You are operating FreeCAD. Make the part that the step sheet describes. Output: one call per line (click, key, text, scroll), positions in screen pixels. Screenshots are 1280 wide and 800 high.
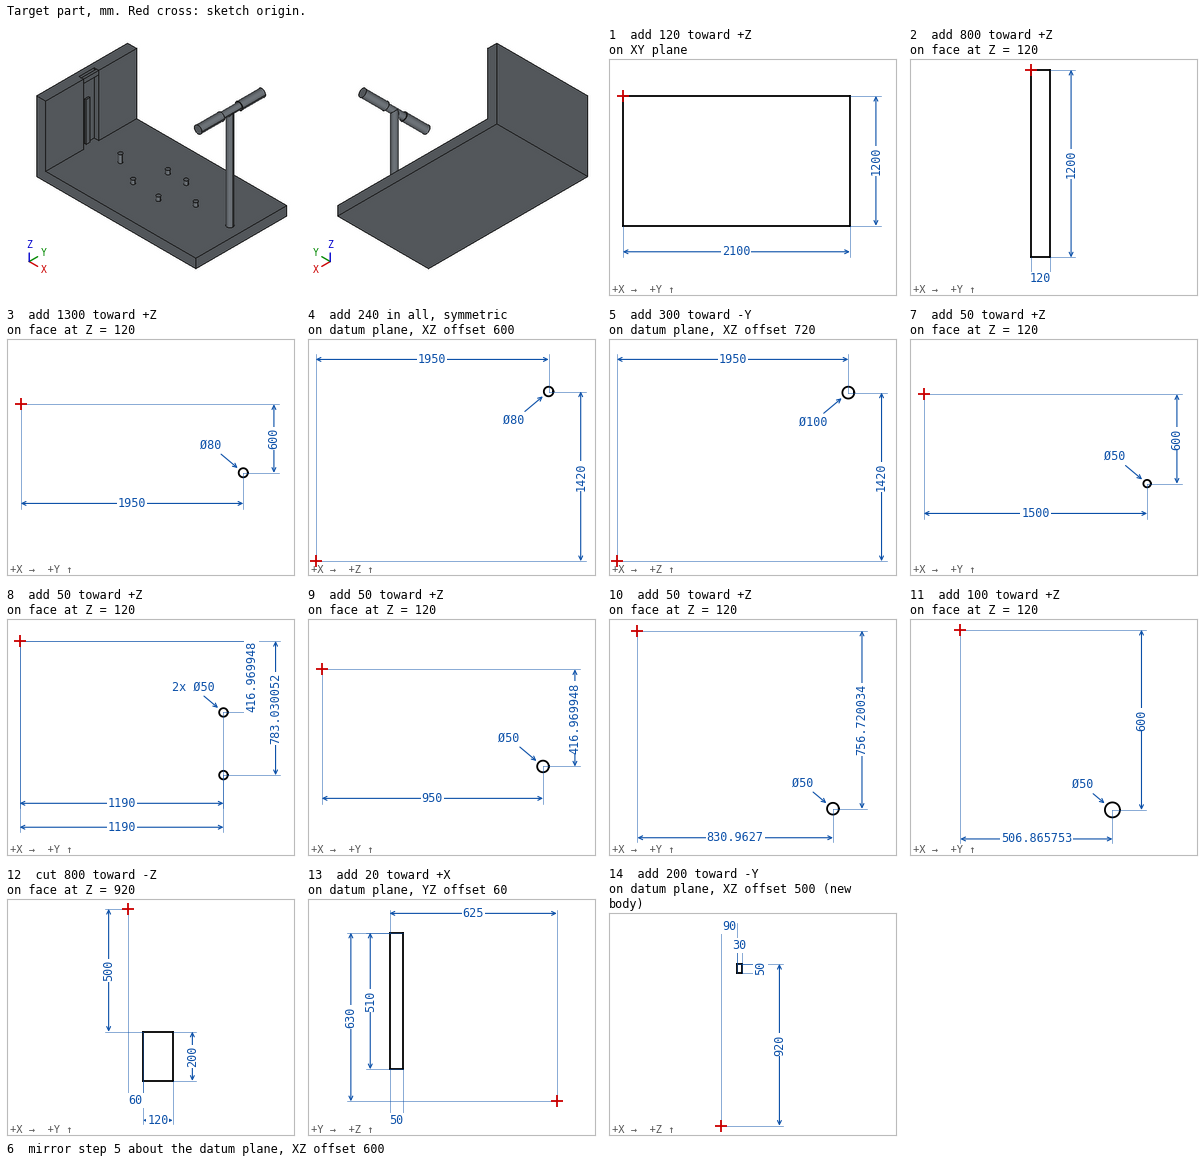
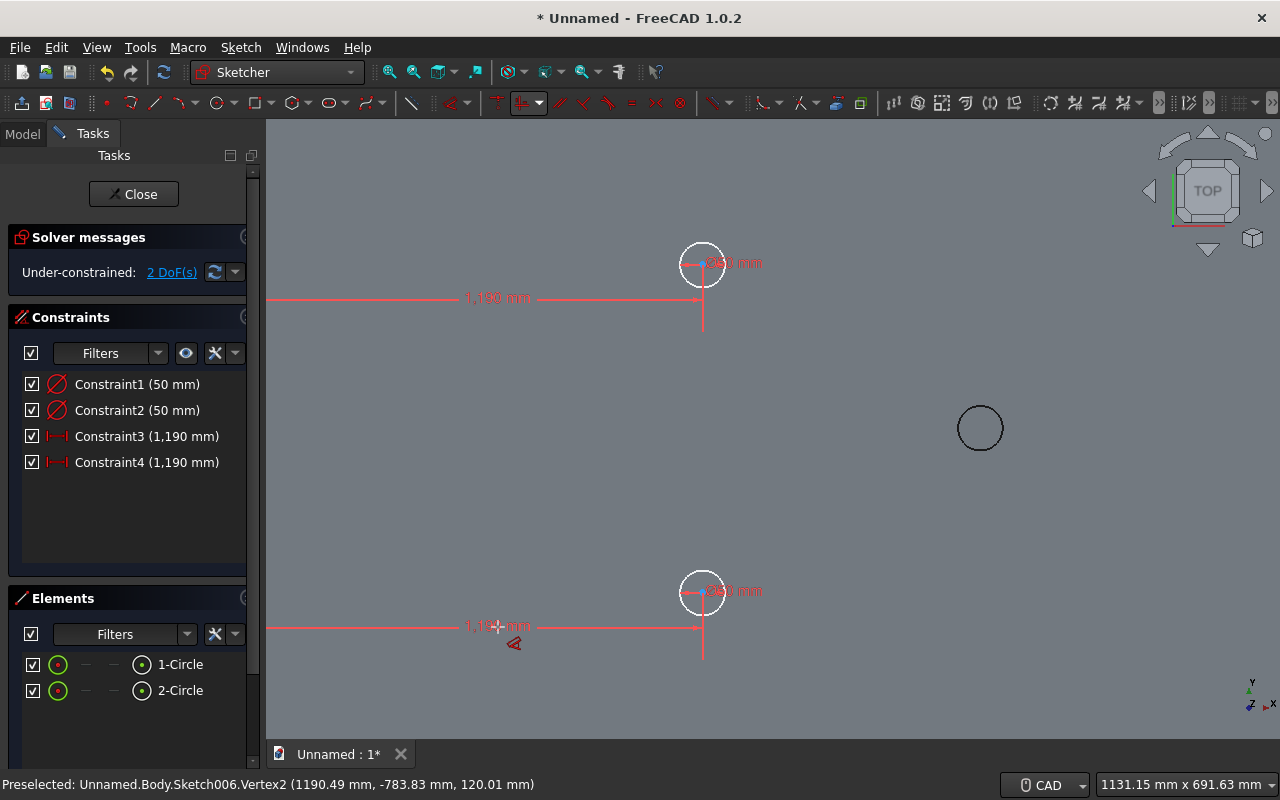
click(703, 265)
click(737, 206)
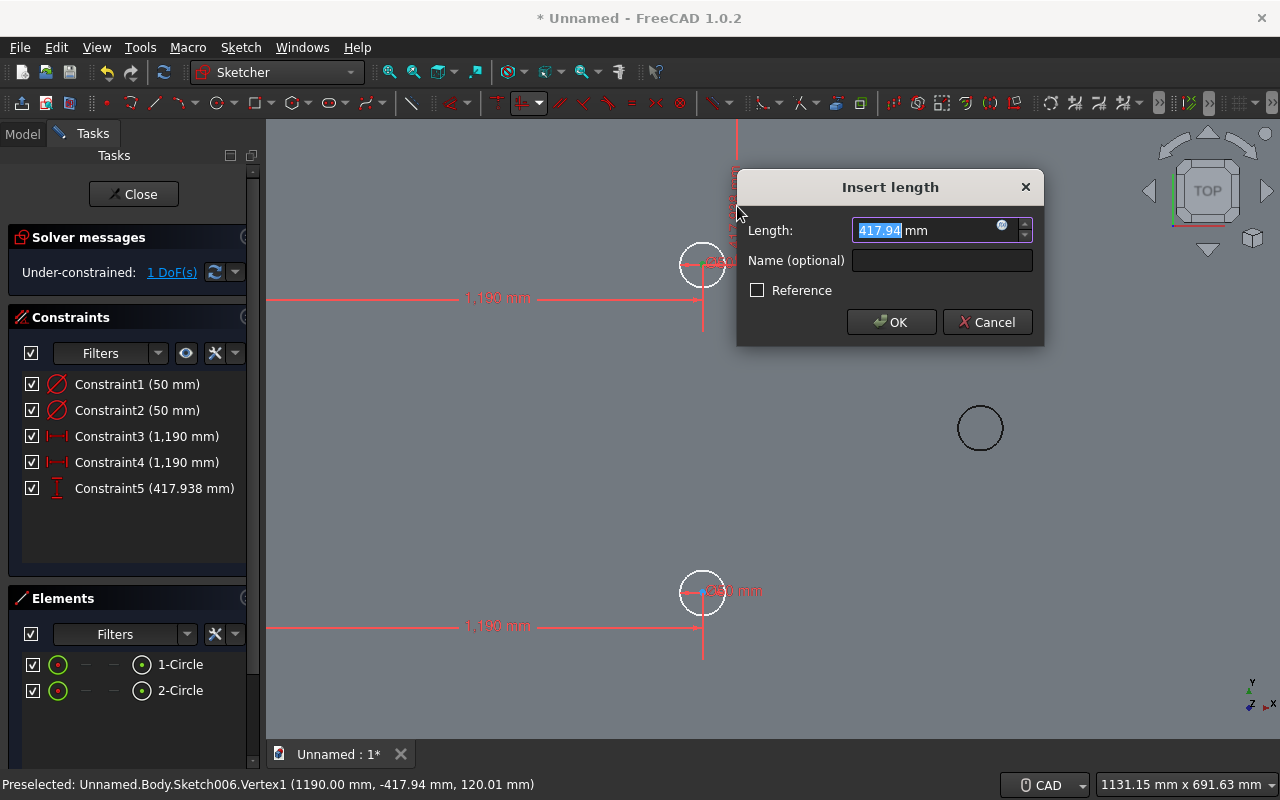
text(416.969948)
key(Return)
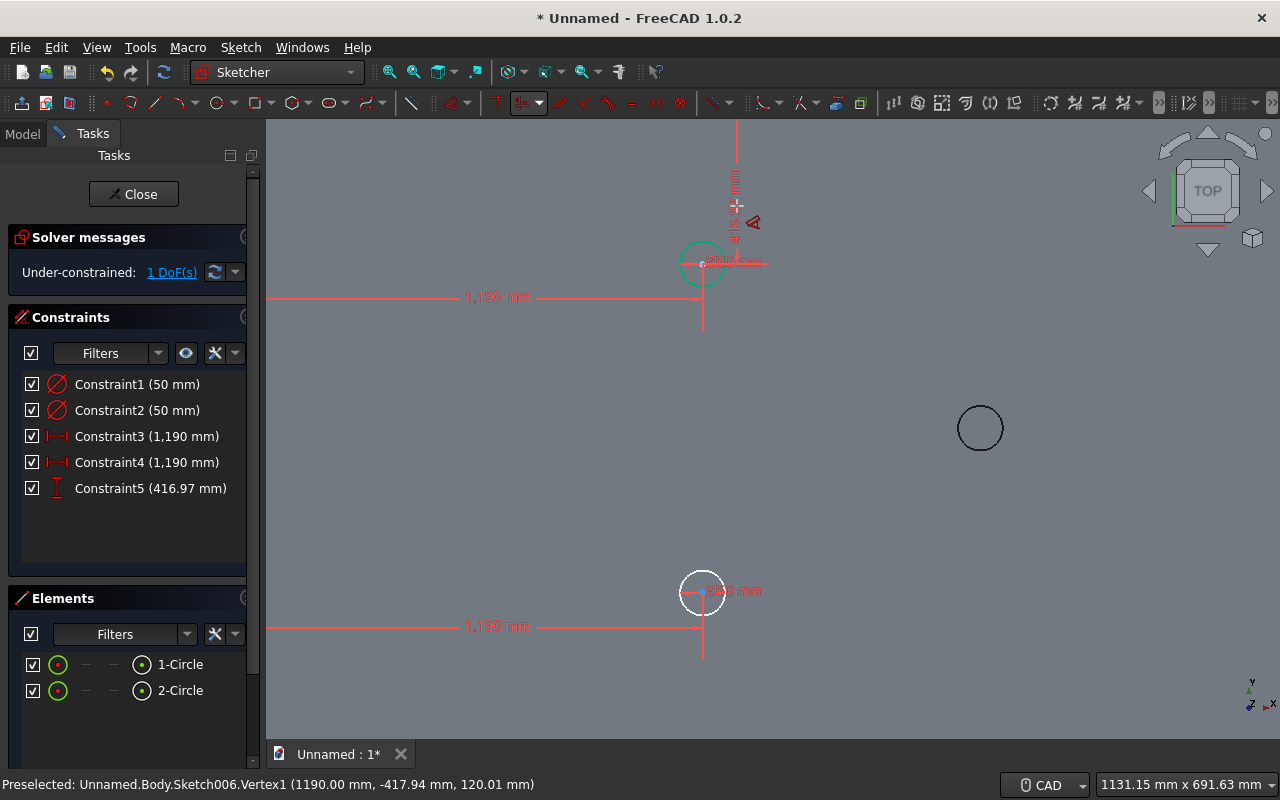
click(703, 593)
click(737, 370)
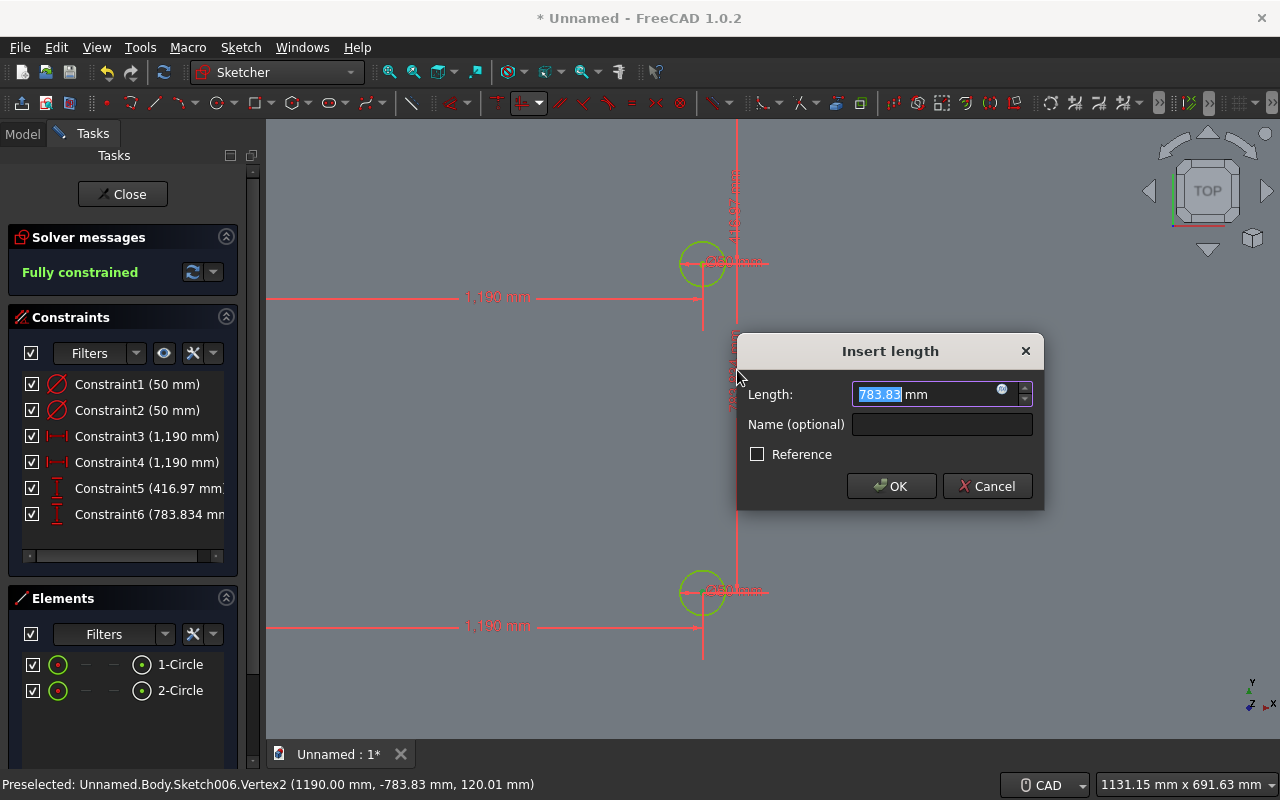
text(783.030052)
key(Return)
key(Escape)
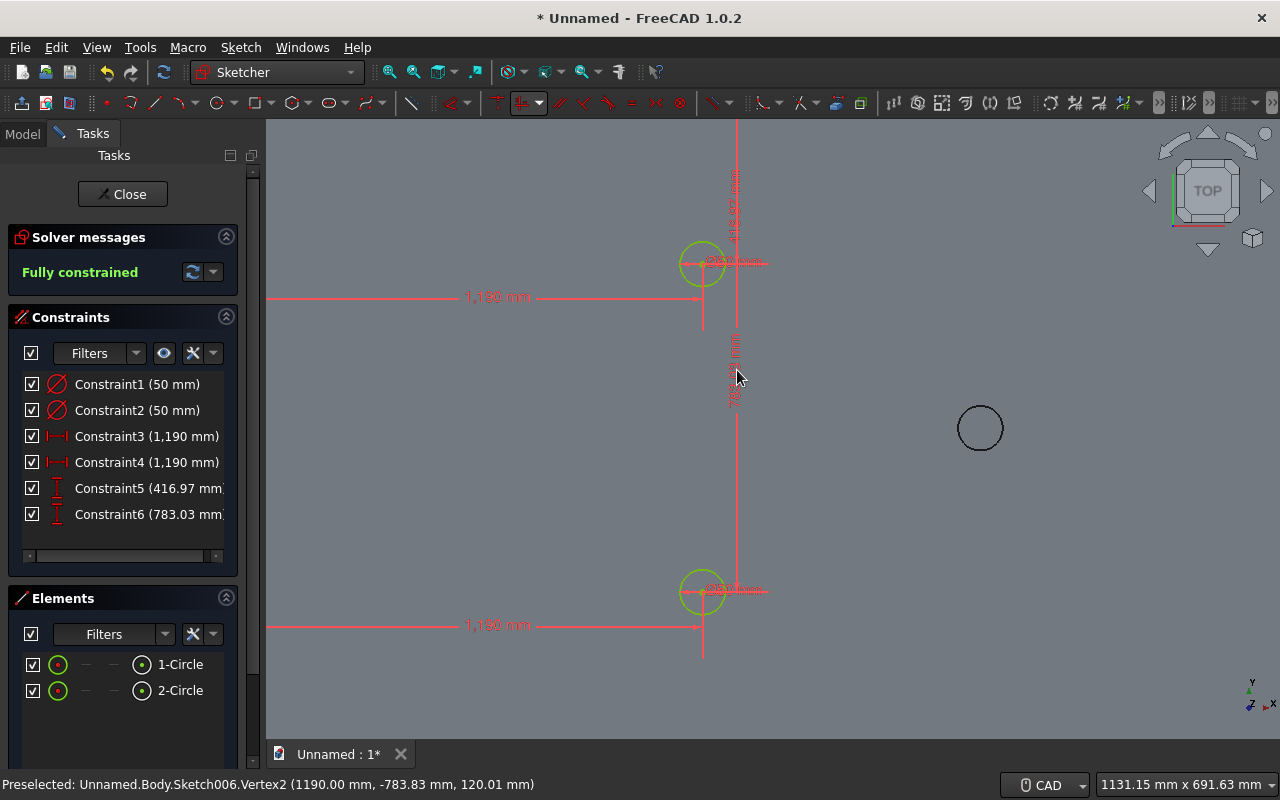
click(123, 194)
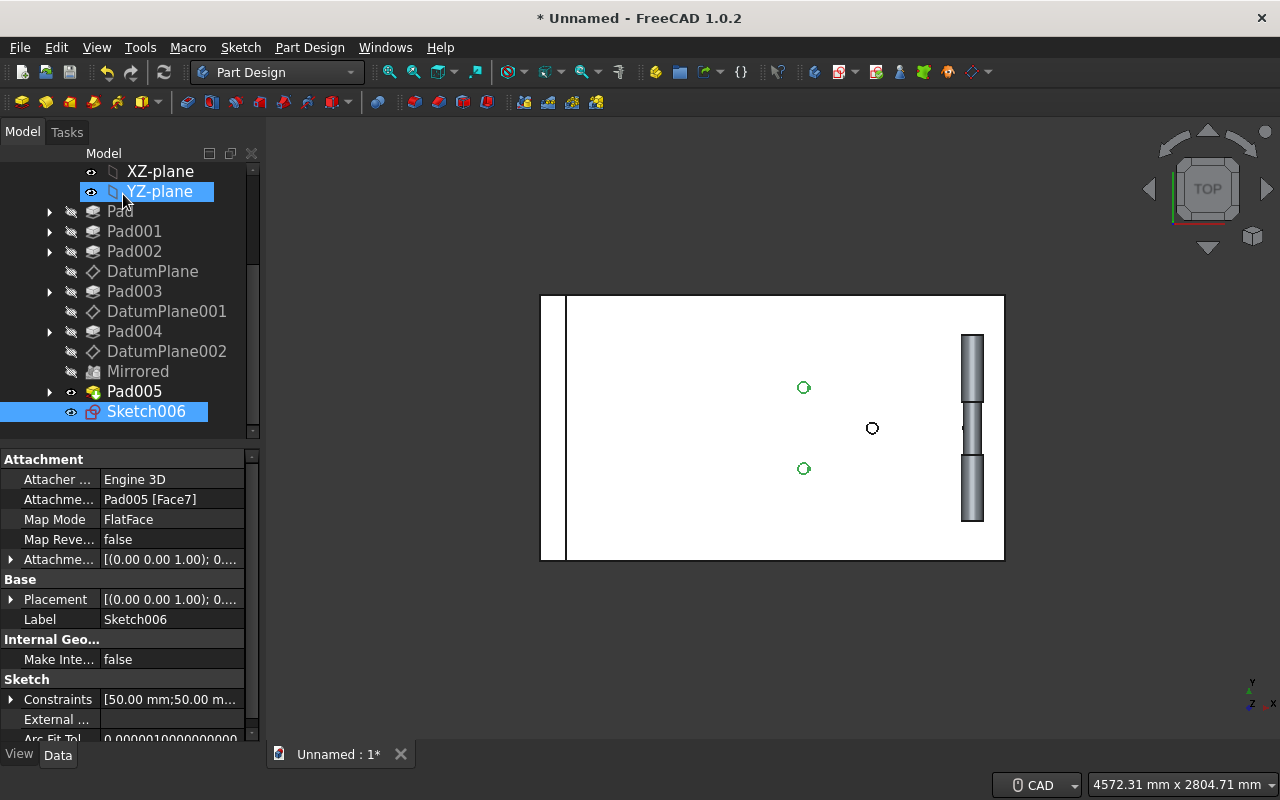
click(22, 102)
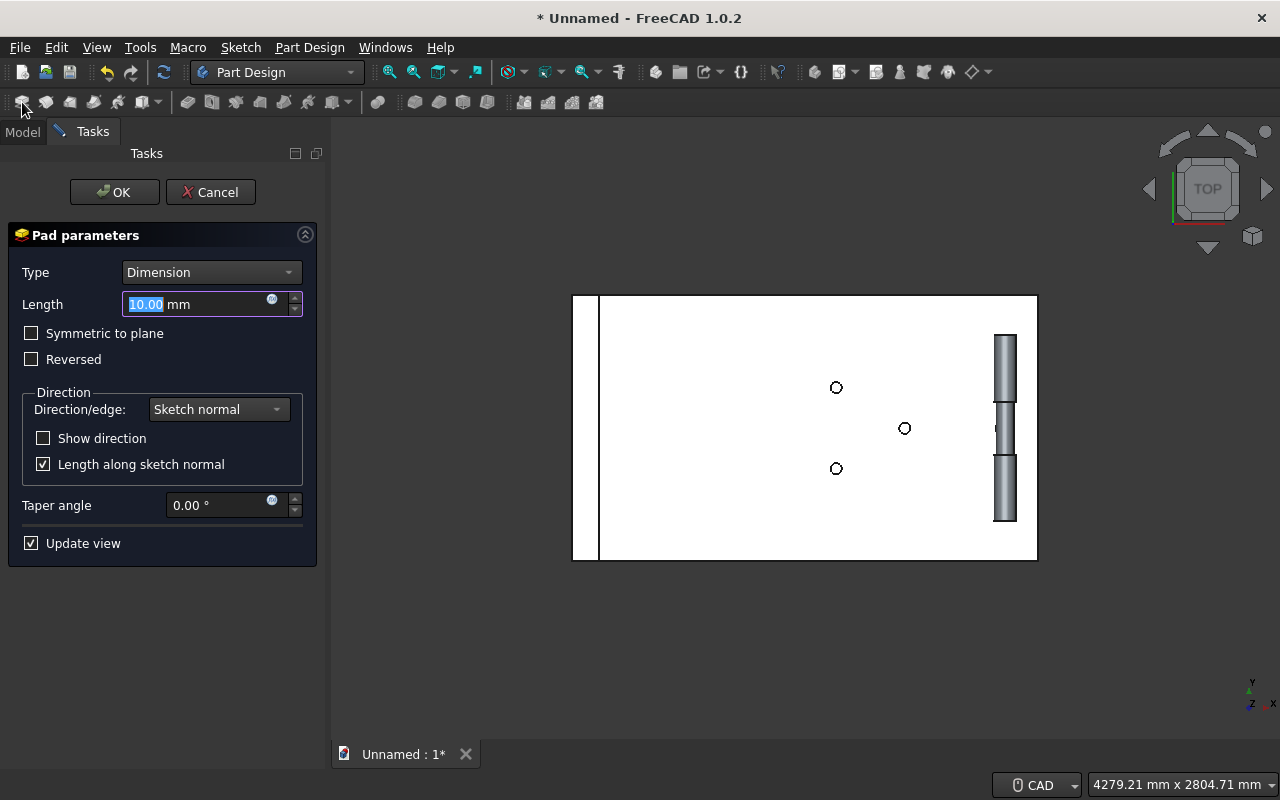
text(50)
key(Tab)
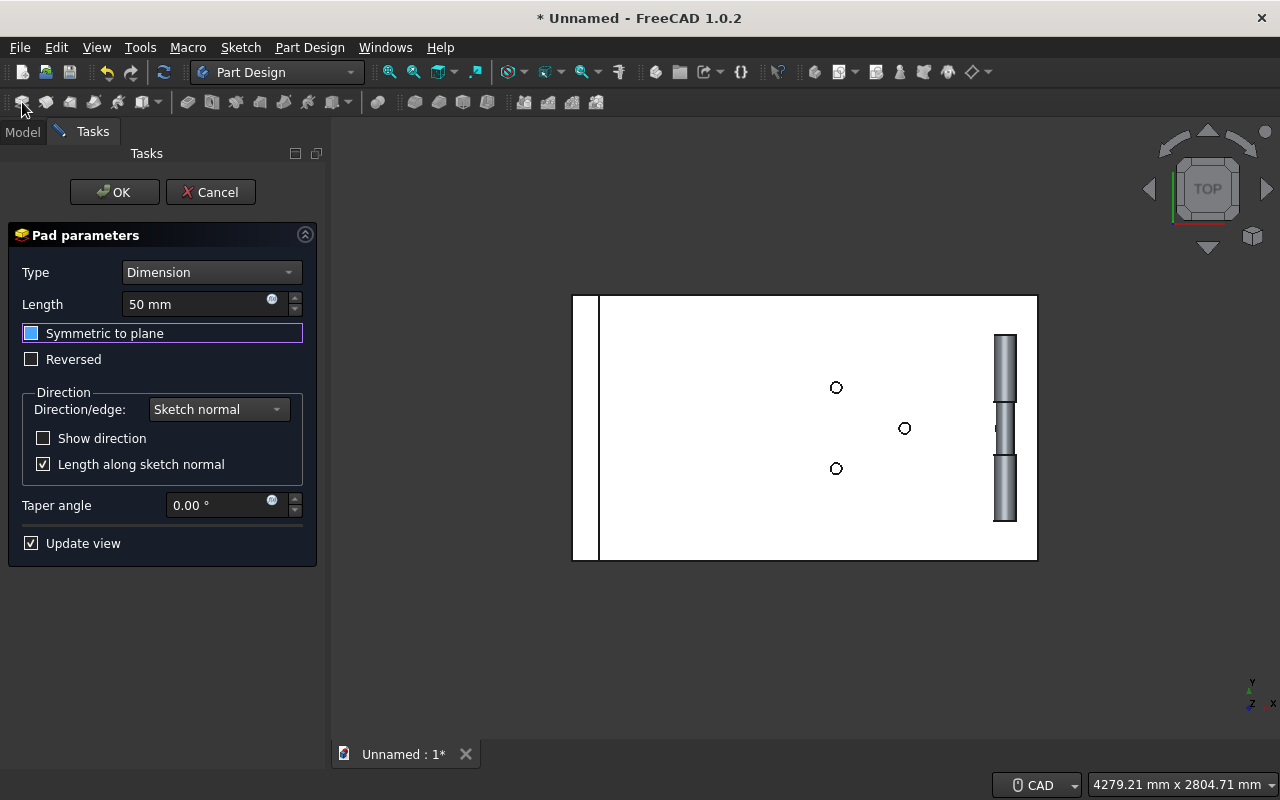
click(115, 192)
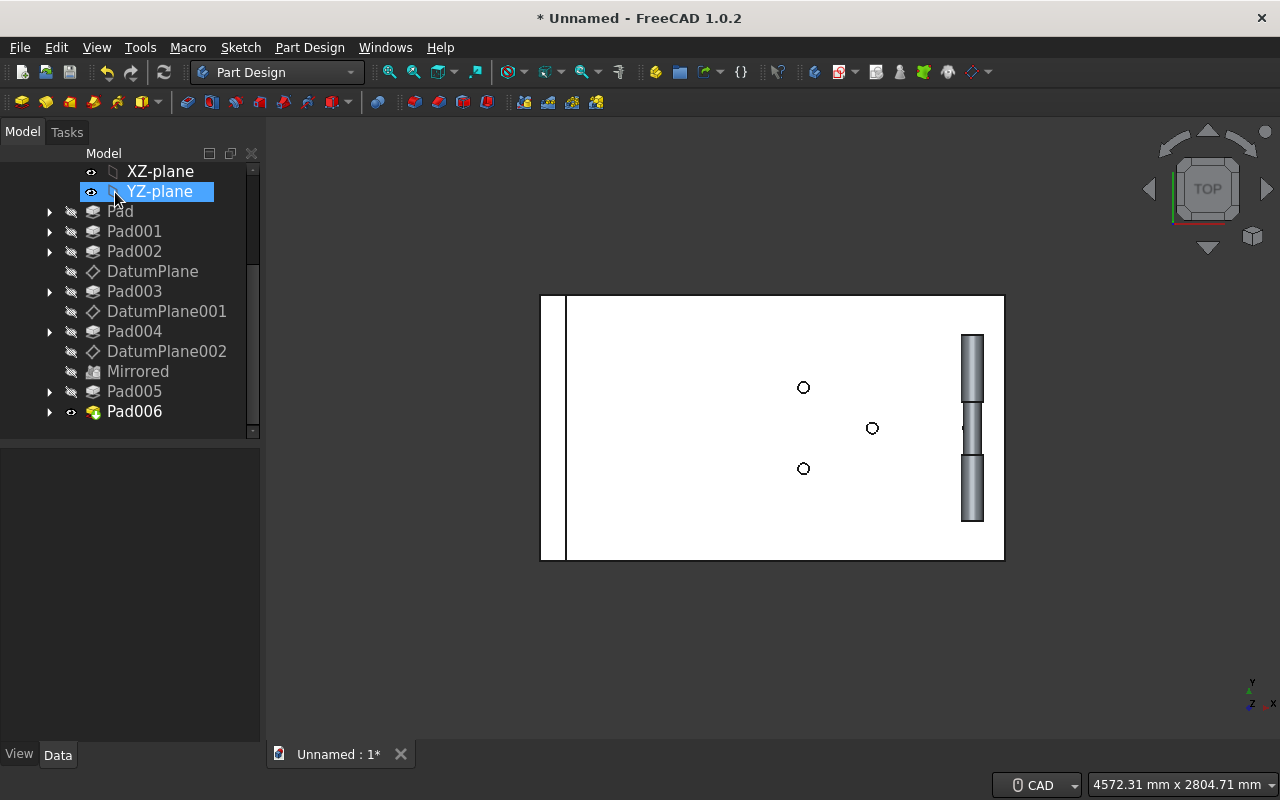
click(660, 389)